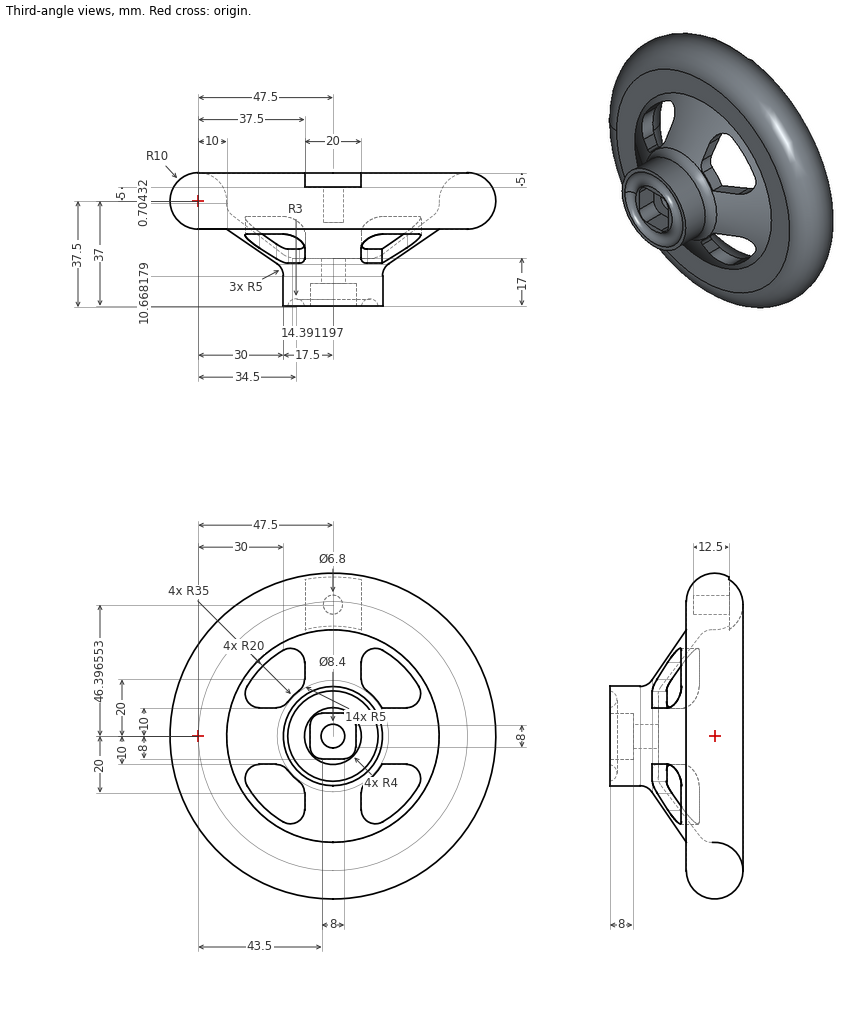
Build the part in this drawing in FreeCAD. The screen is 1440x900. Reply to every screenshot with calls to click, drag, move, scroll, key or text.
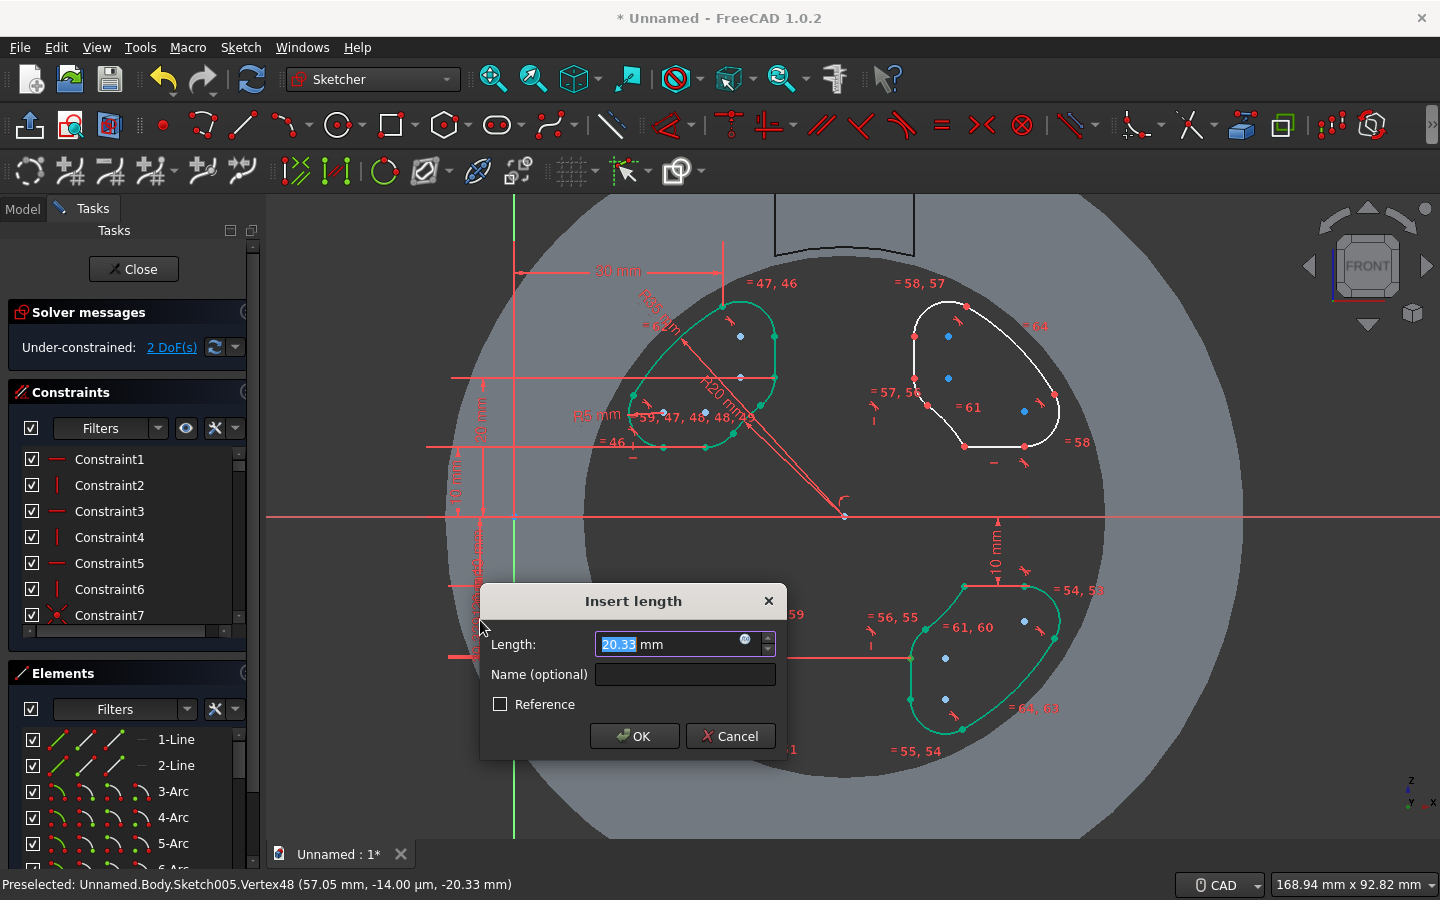
text(20)
key(Return)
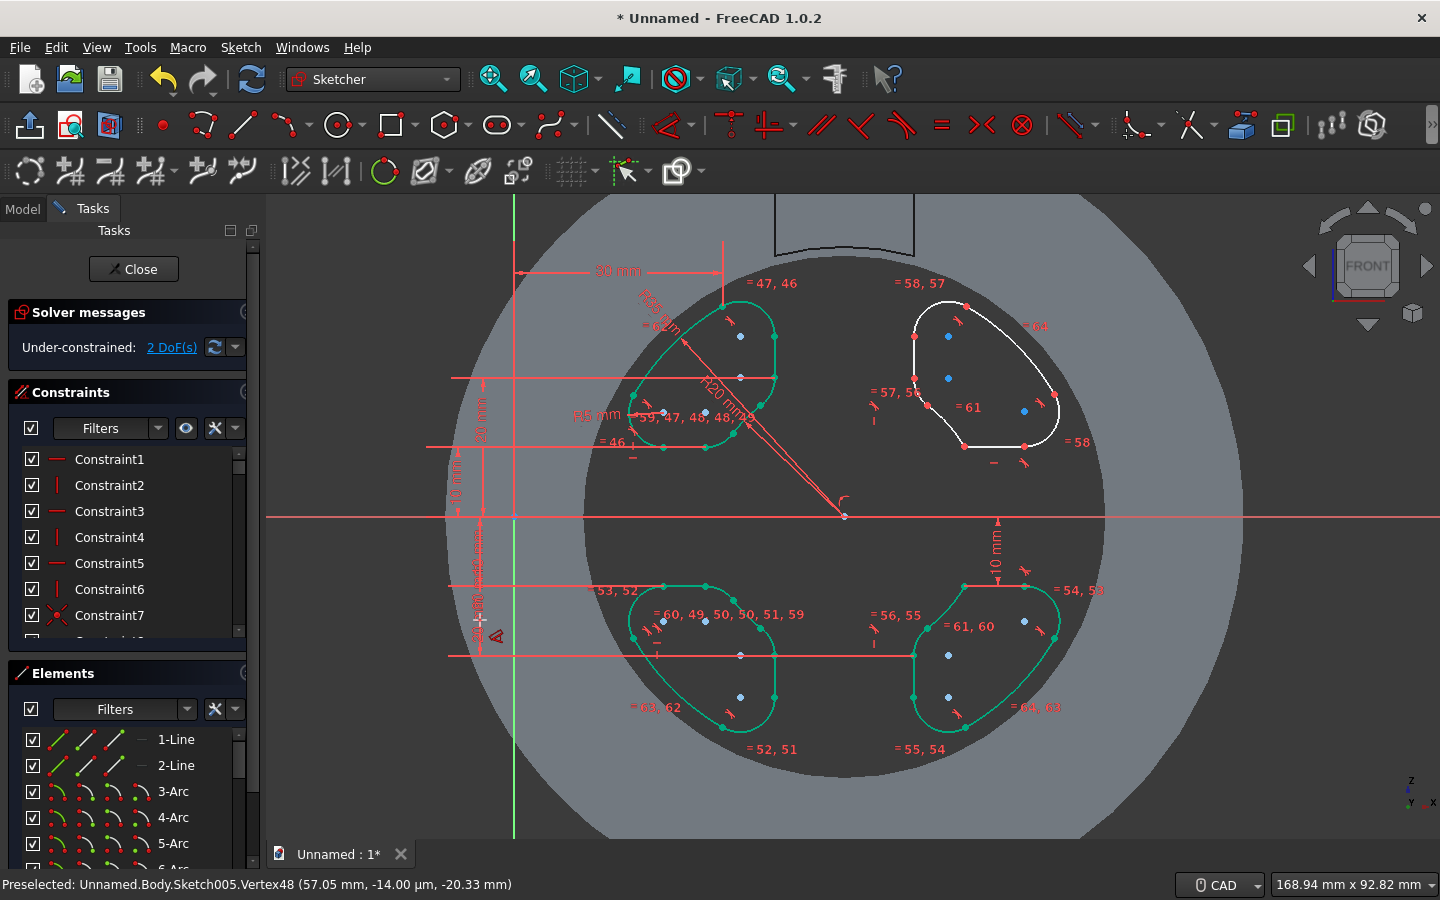
click(1024, 447)
click(480, 498)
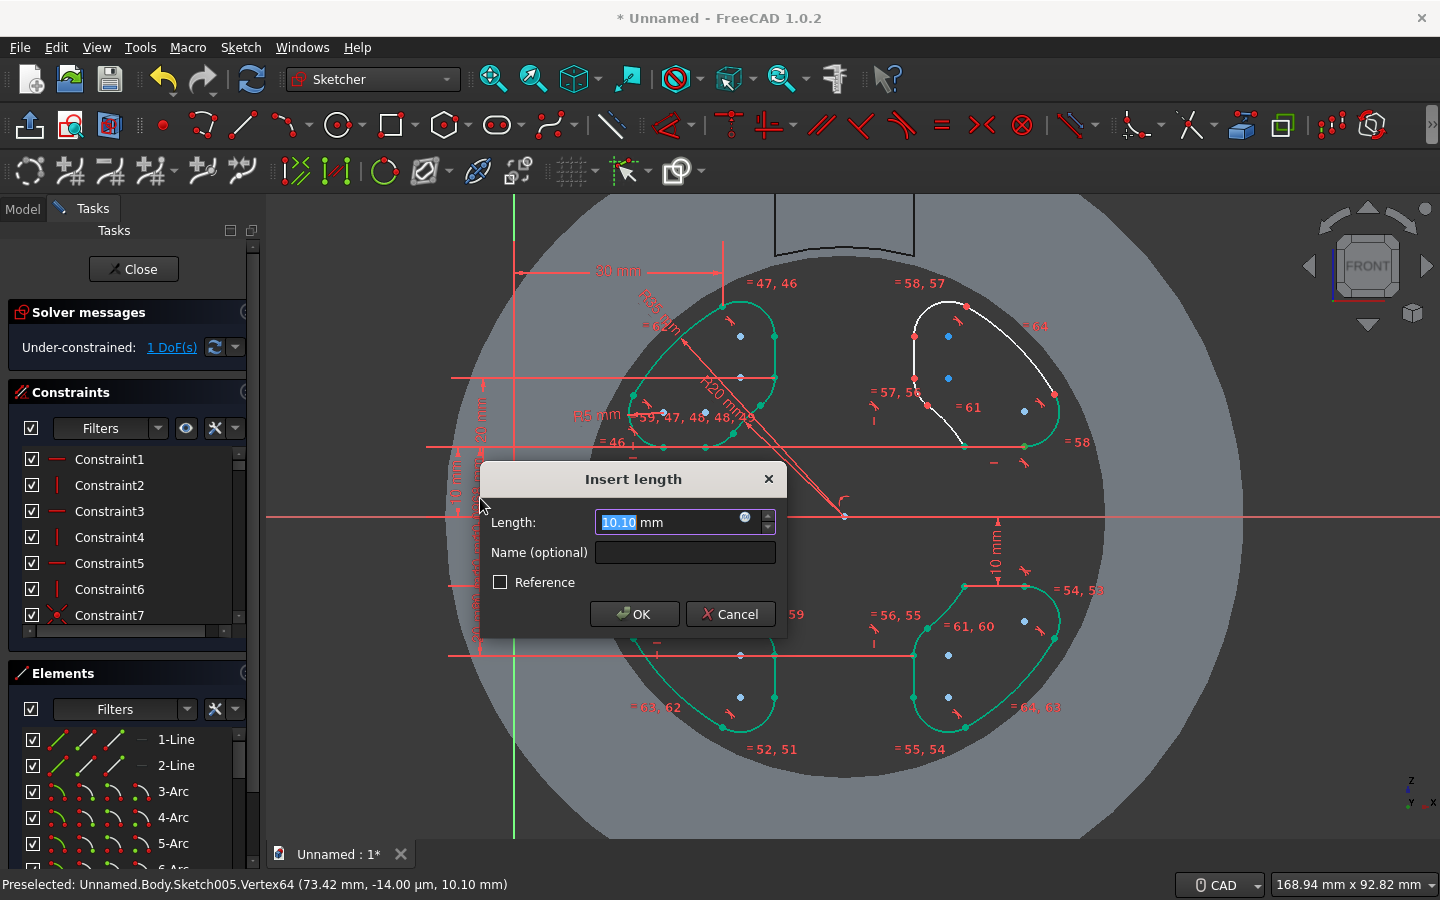
text(10)
key(Return)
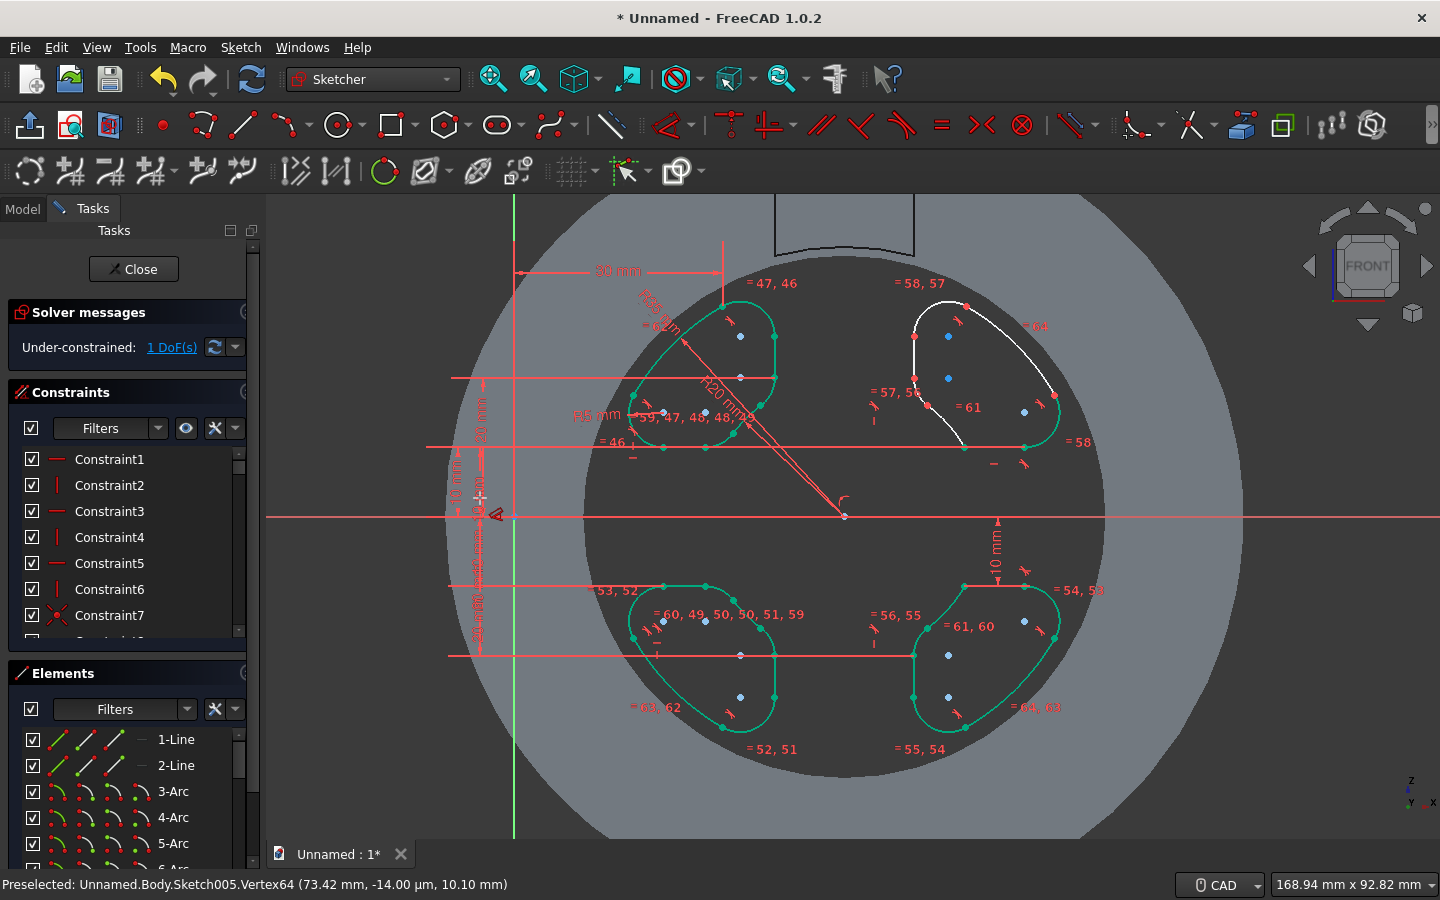
click(914, 378)
click(480, 447)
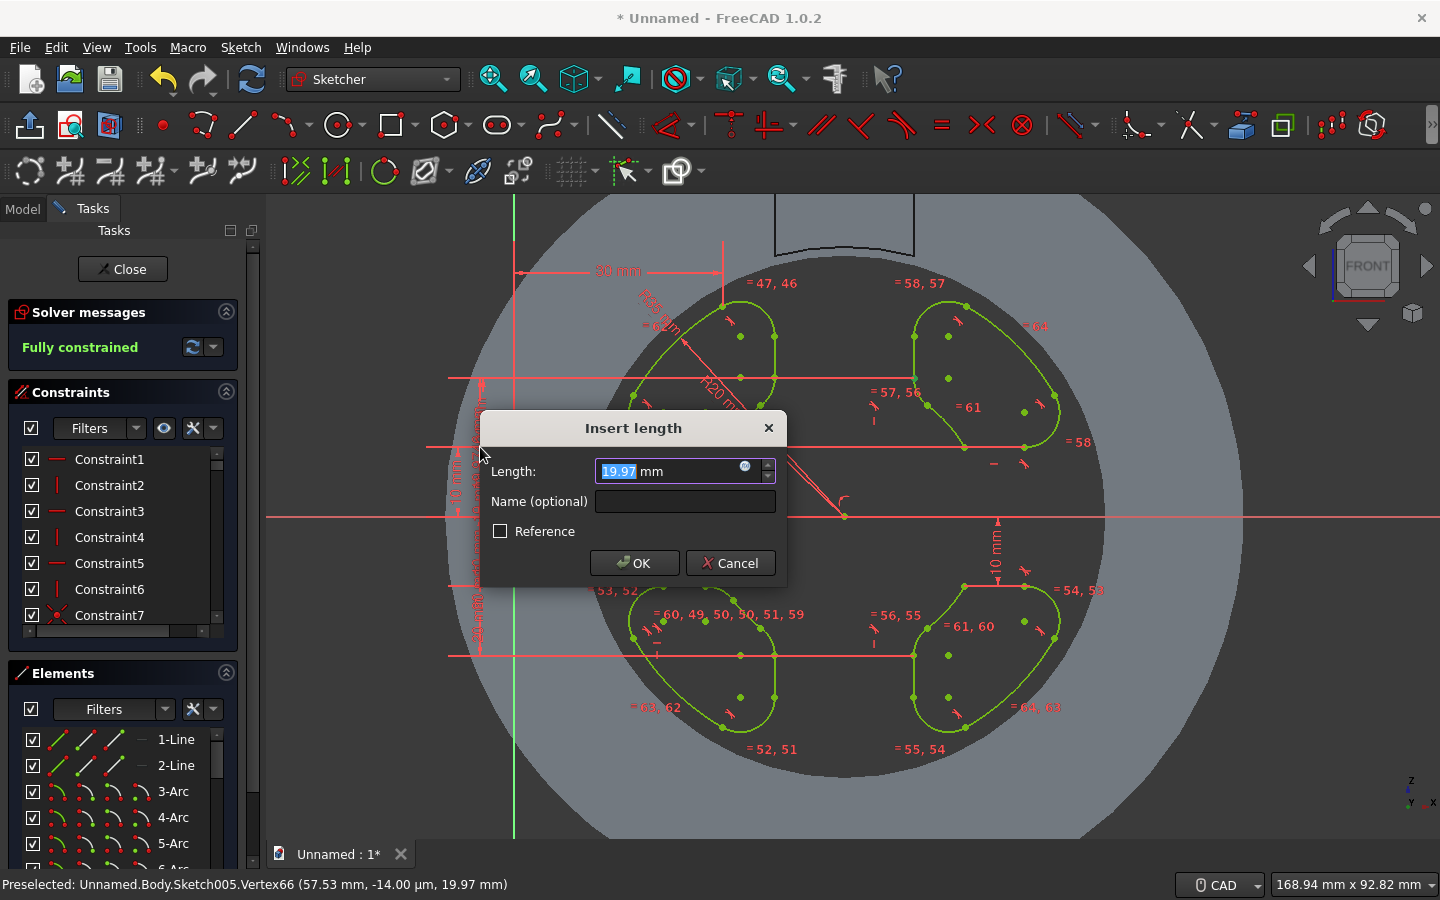
text(20)
key(Return)
key(Escape)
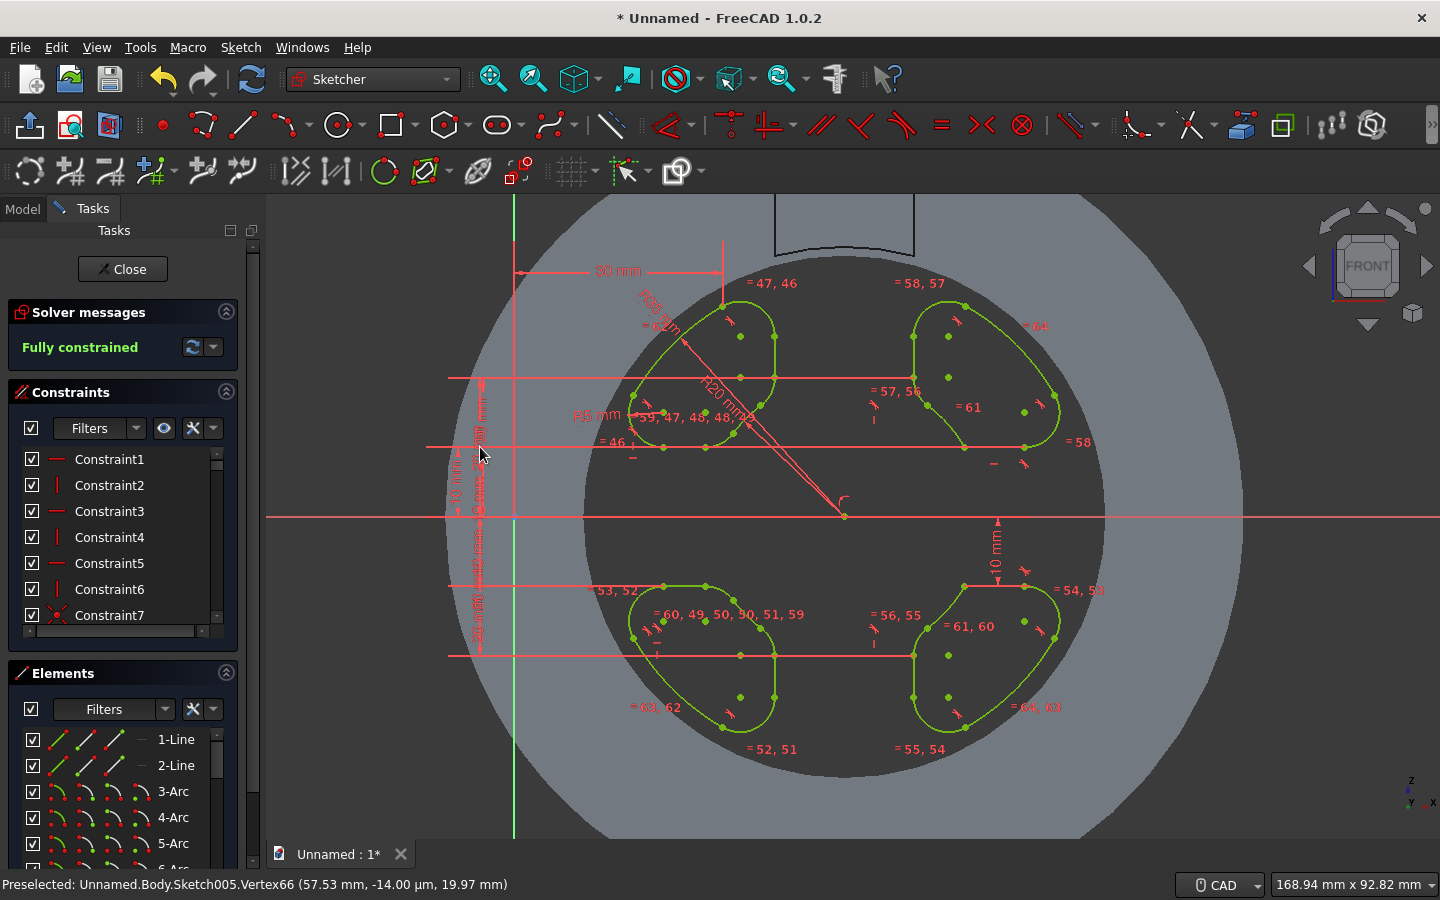
click(123, 269)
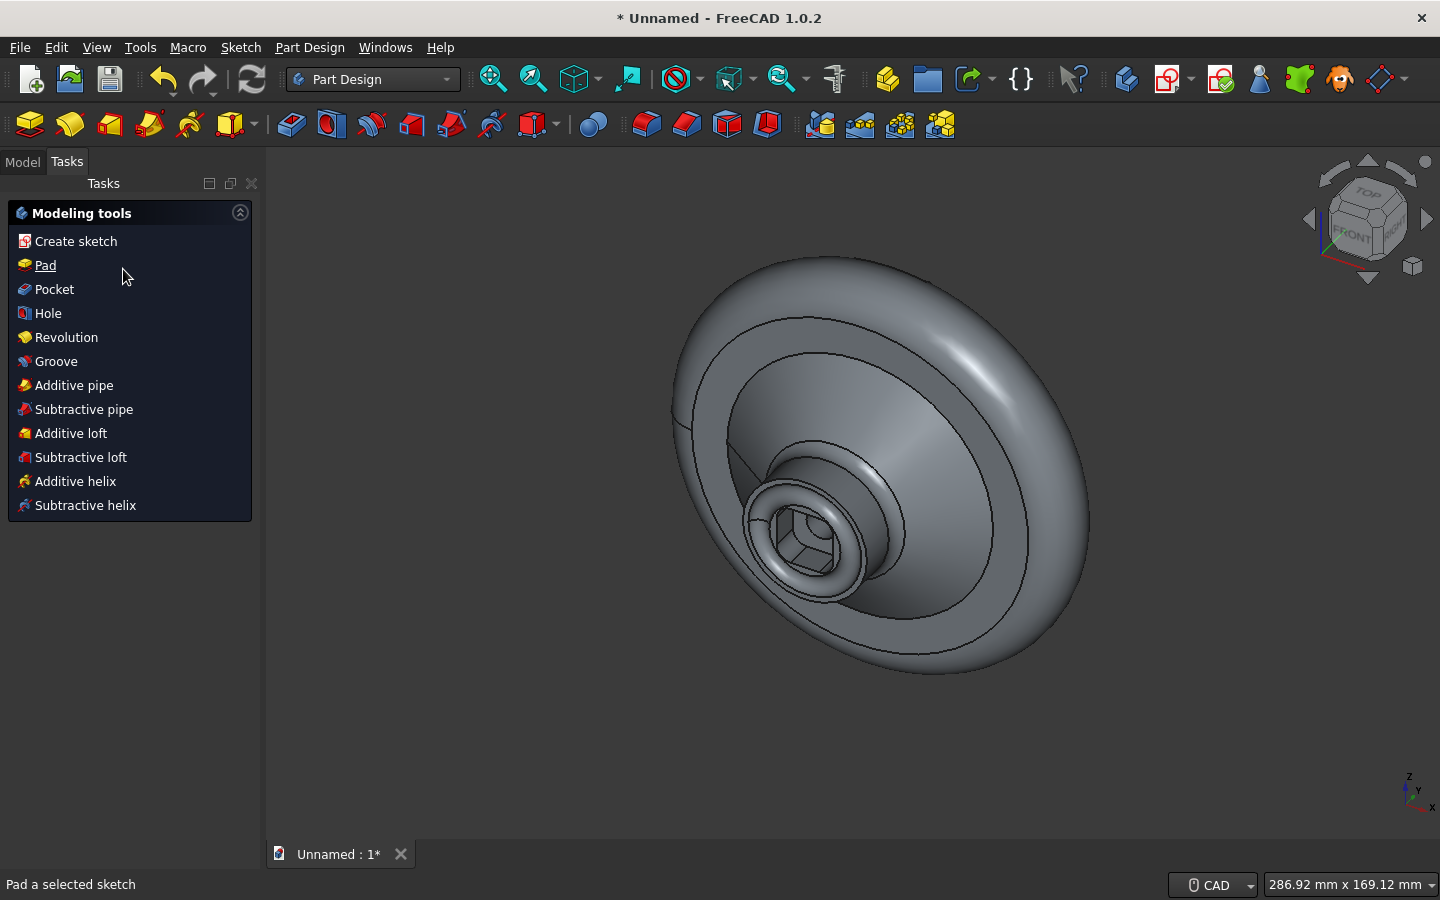
click(292, 124)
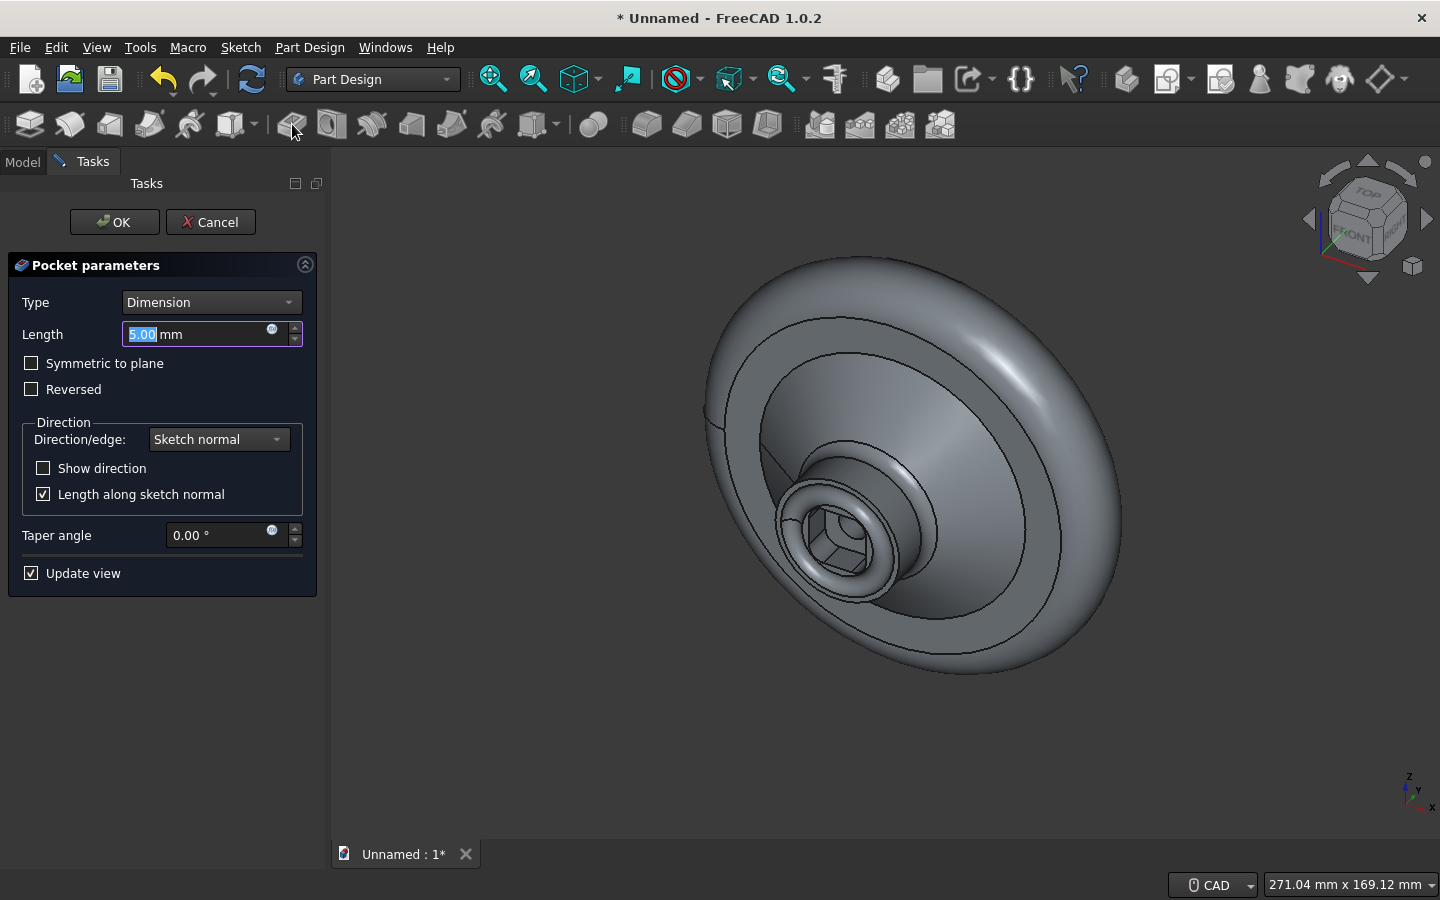
click(212, 302)